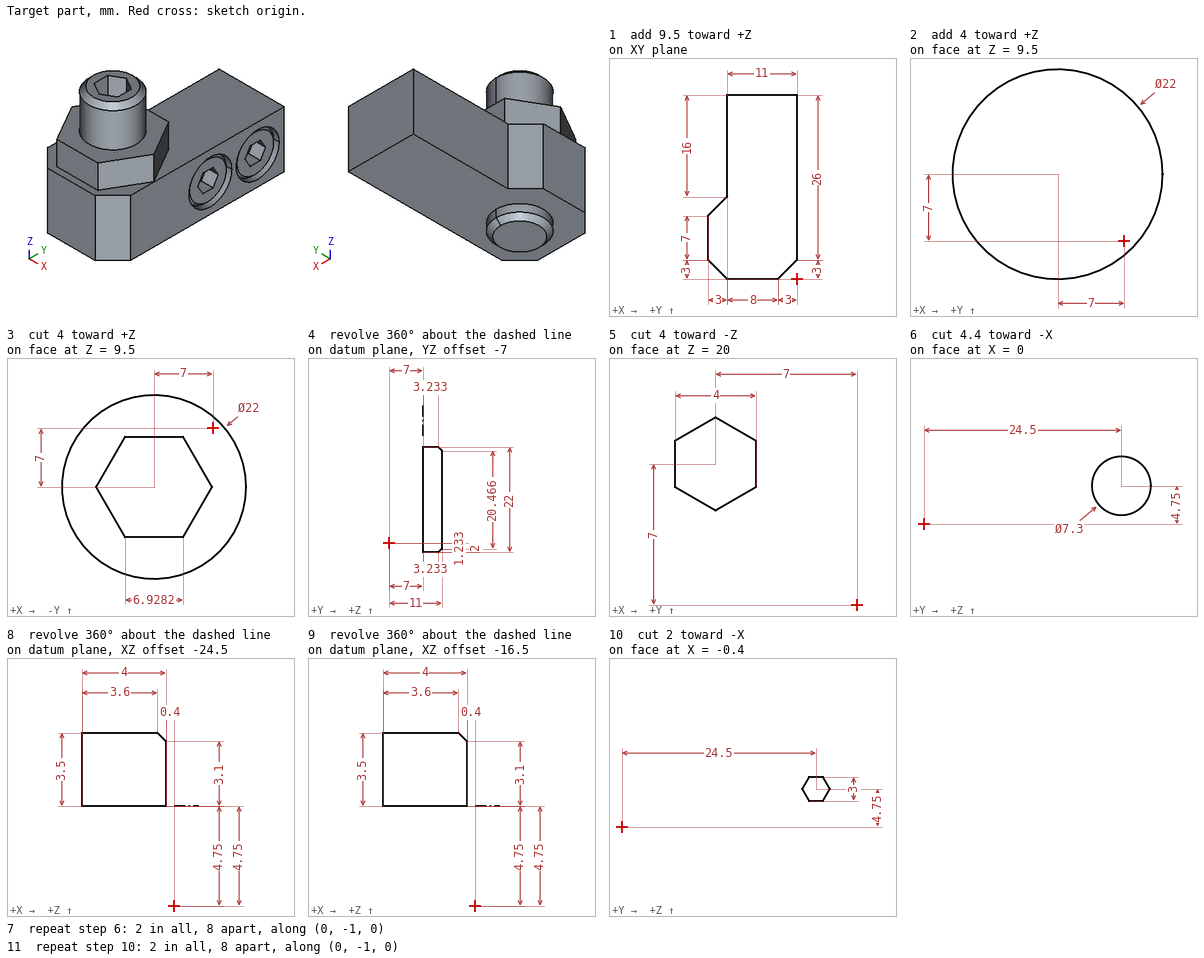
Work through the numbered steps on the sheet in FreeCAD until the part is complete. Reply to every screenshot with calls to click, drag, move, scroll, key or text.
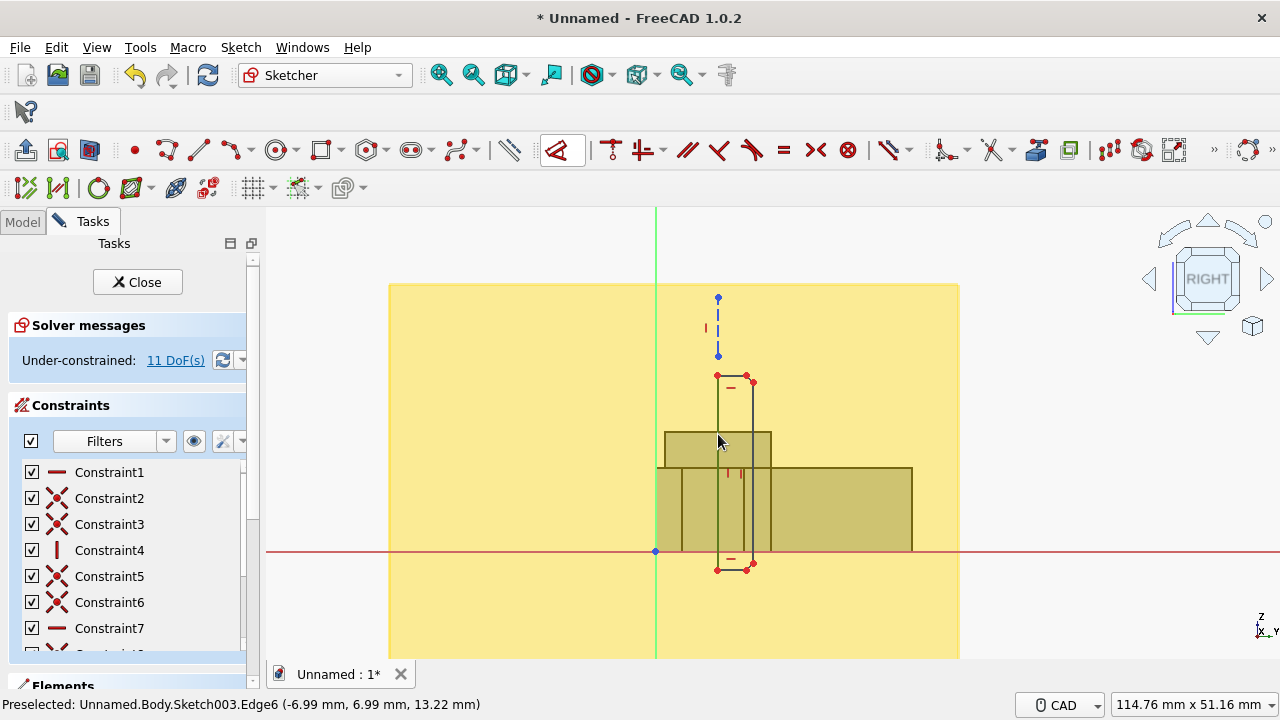
key(i)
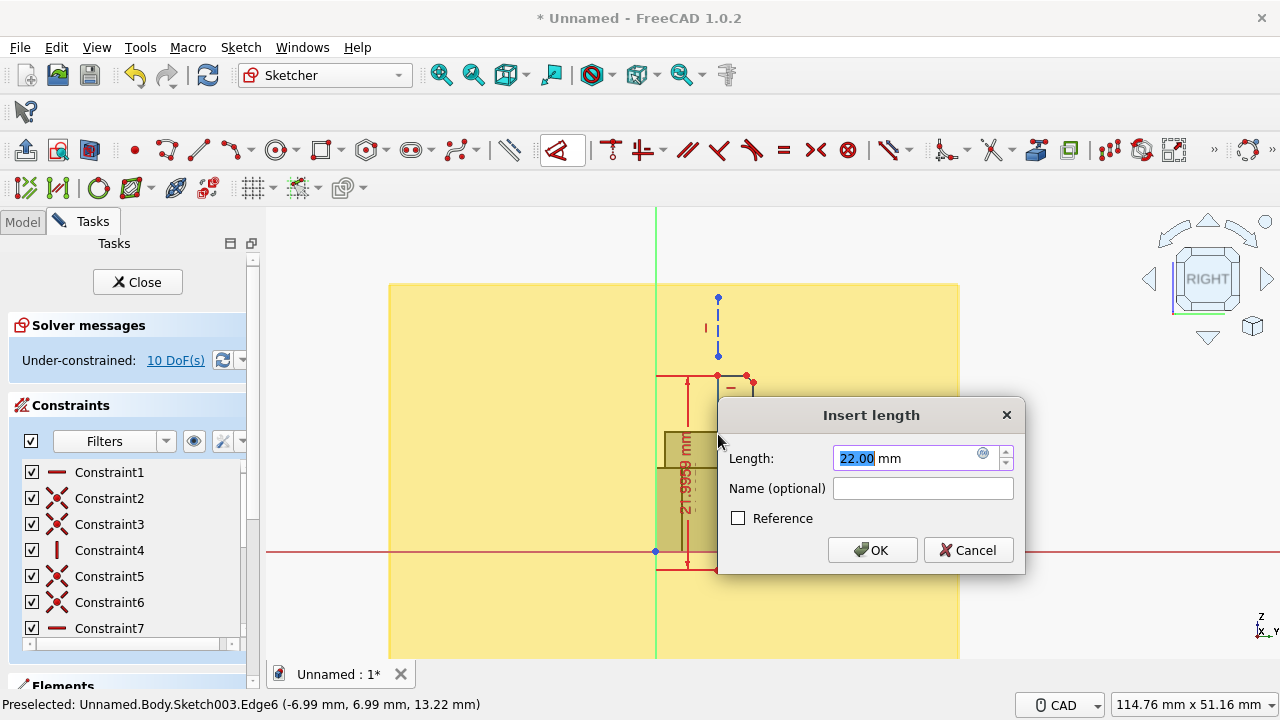
text(22)
key(Return)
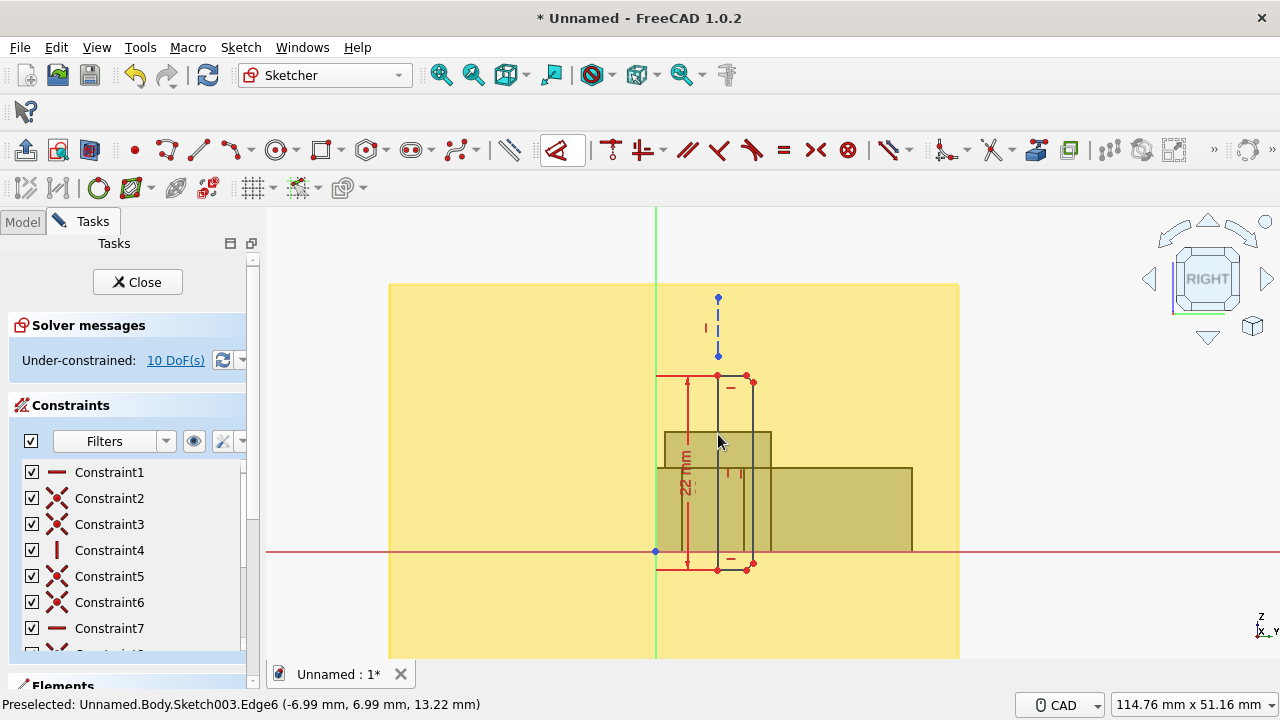
click(718, 570)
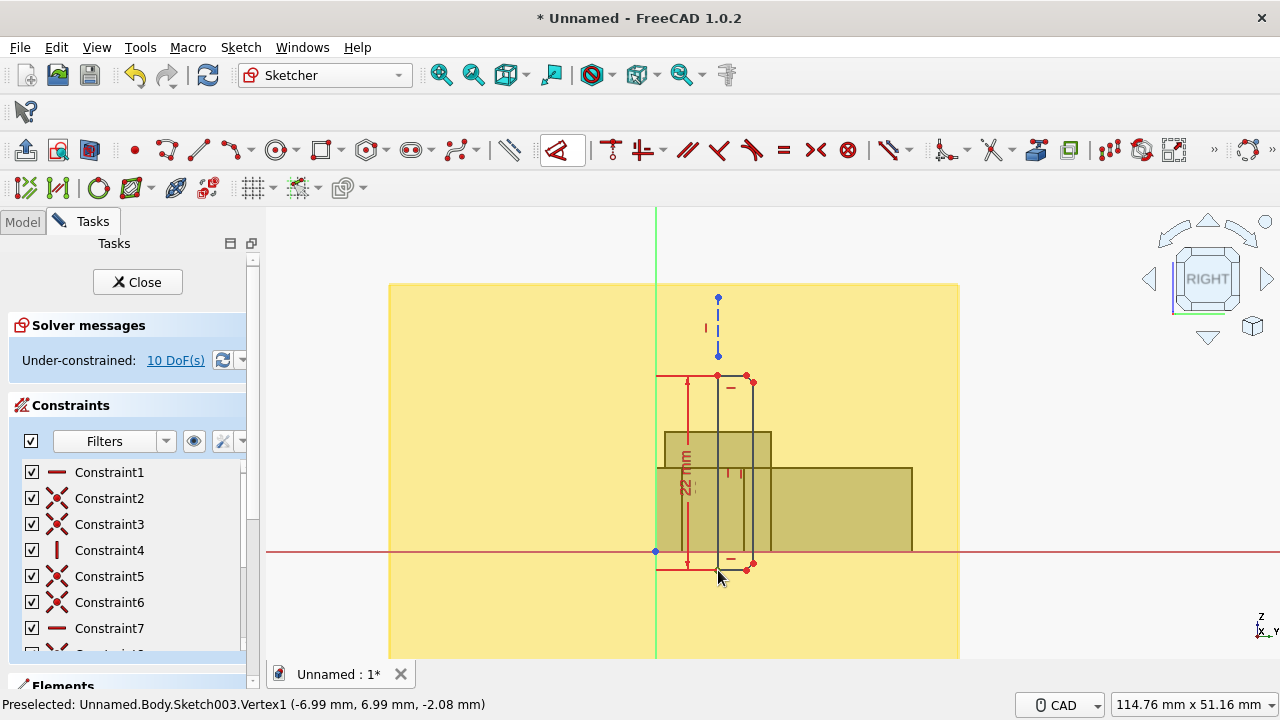
key(l)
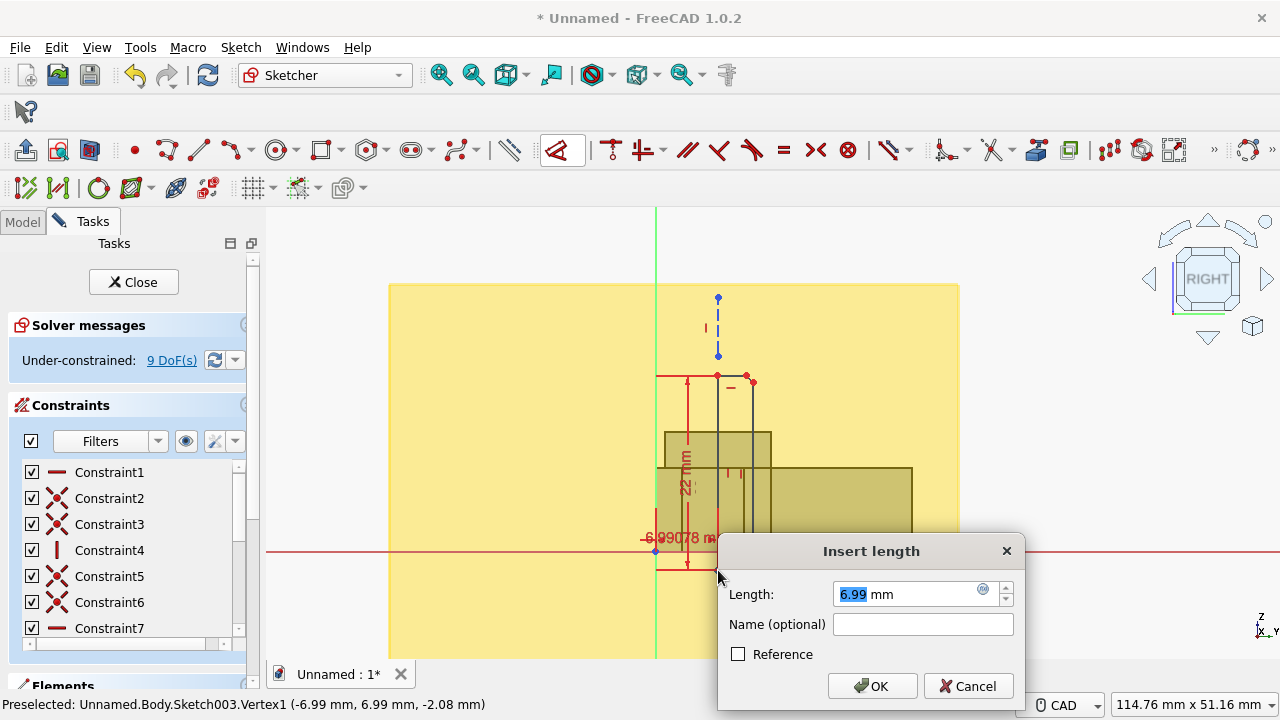
text(7)
key(Return)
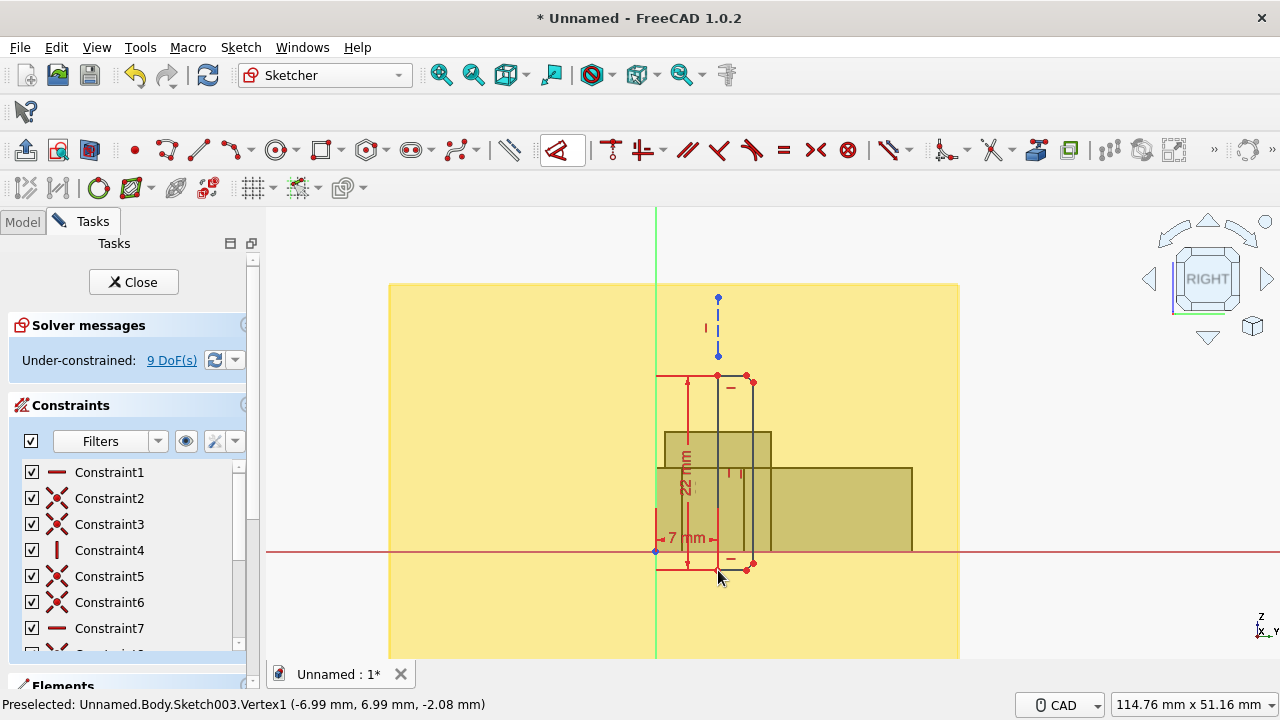
scroll(718, 570, up, 5)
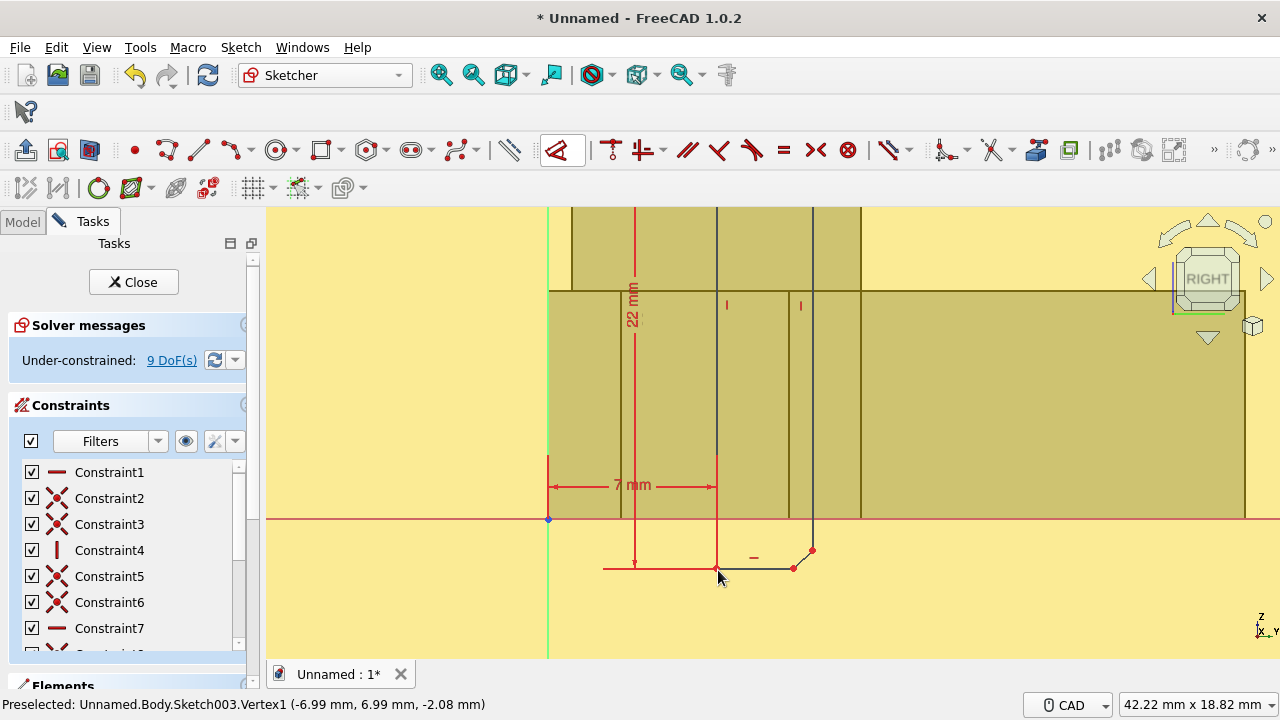
click(717, 569)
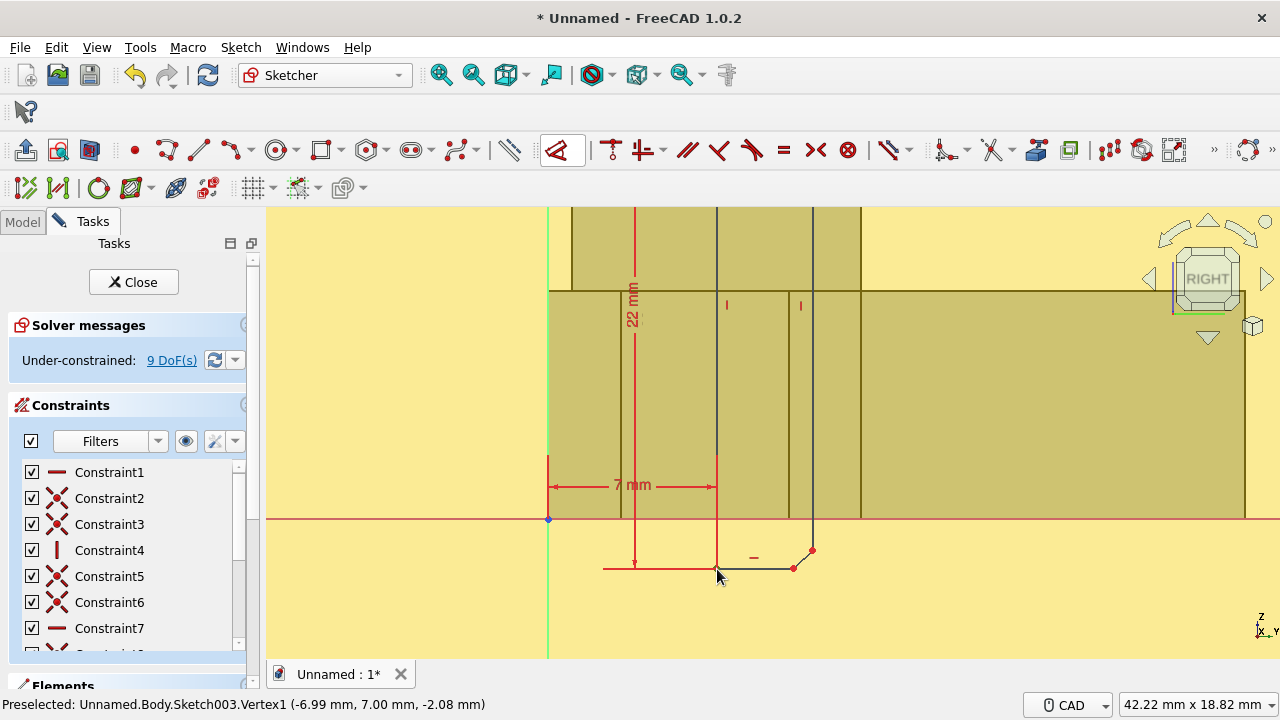
key(i)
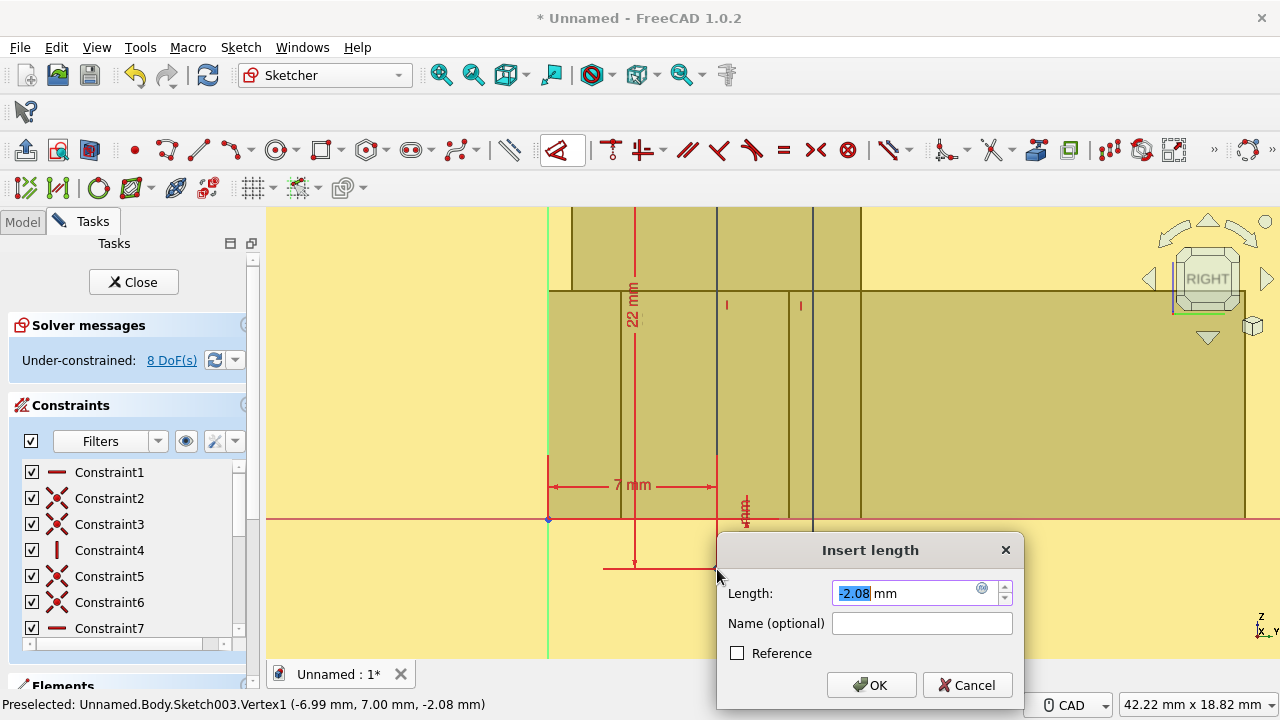
text(-2)
key(Return)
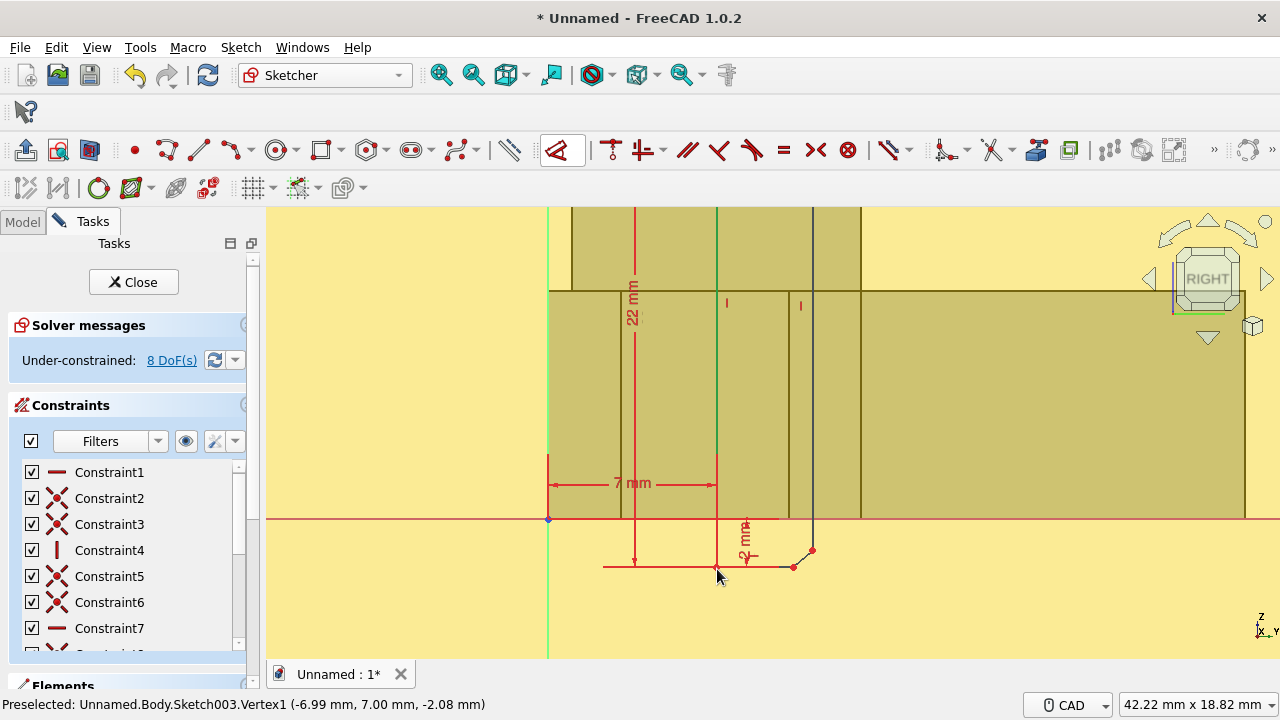
scroll(718, 570, down, 5)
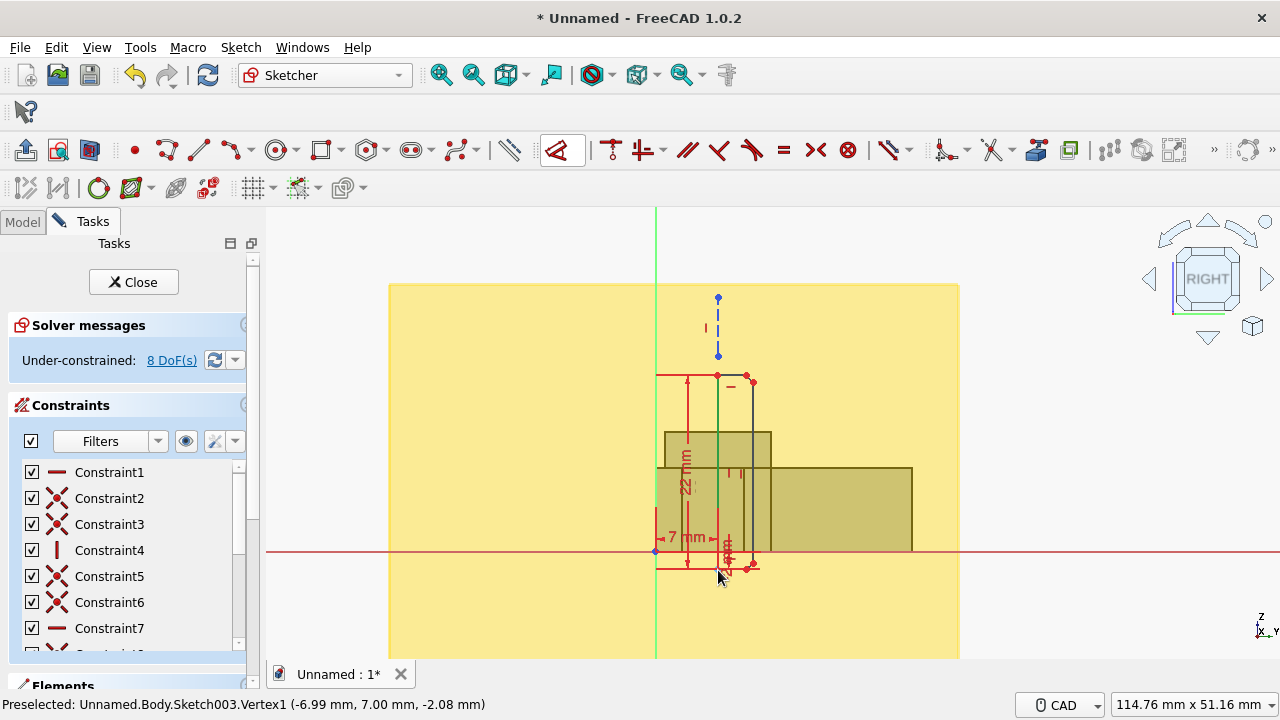
click(718, 357)